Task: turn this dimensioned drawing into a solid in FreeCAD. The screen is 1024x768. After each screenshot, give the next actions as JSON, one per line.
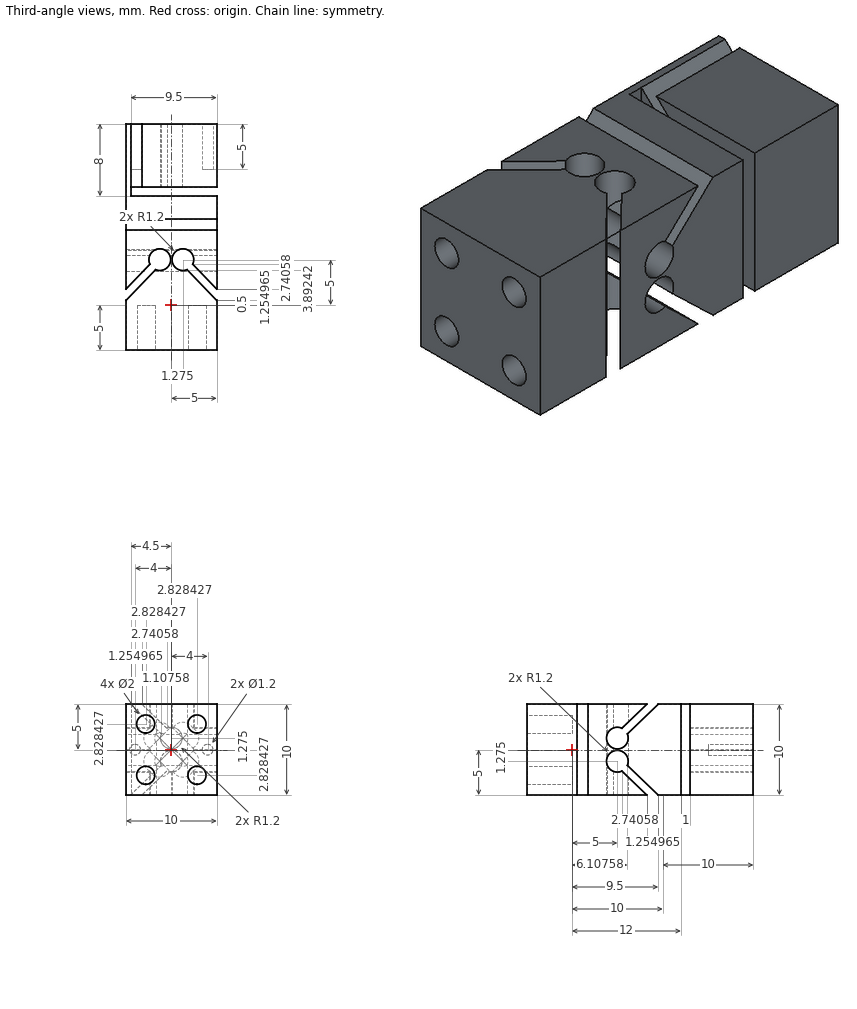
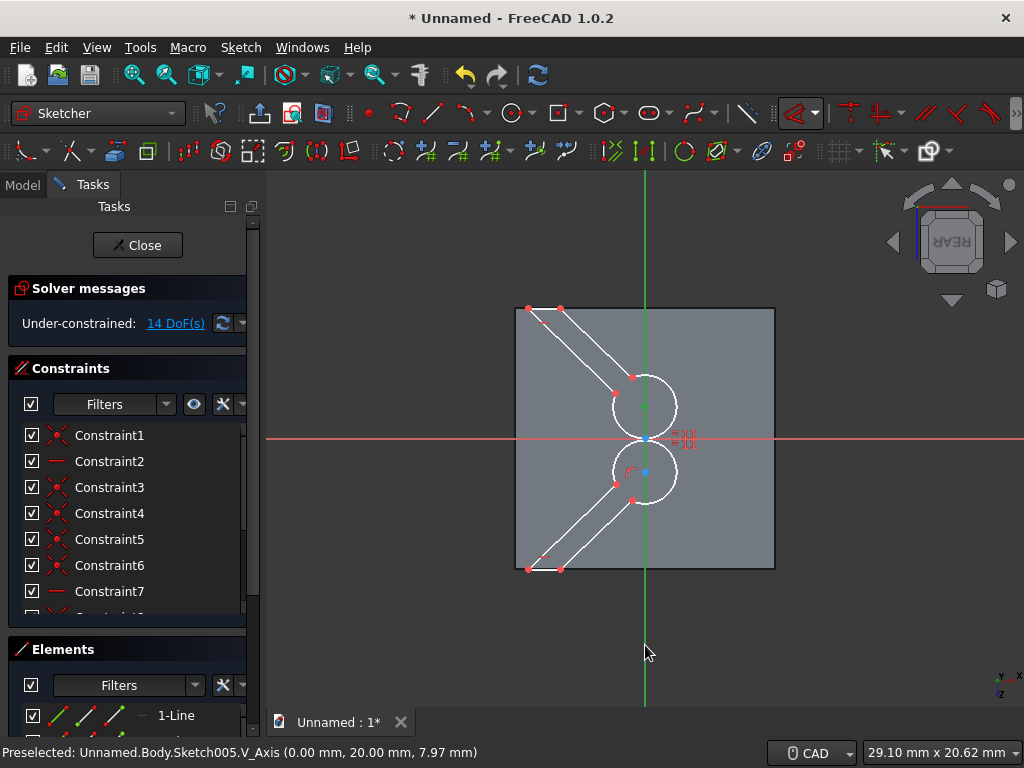
{"action": "left_click", "coordinate": [850, 114]}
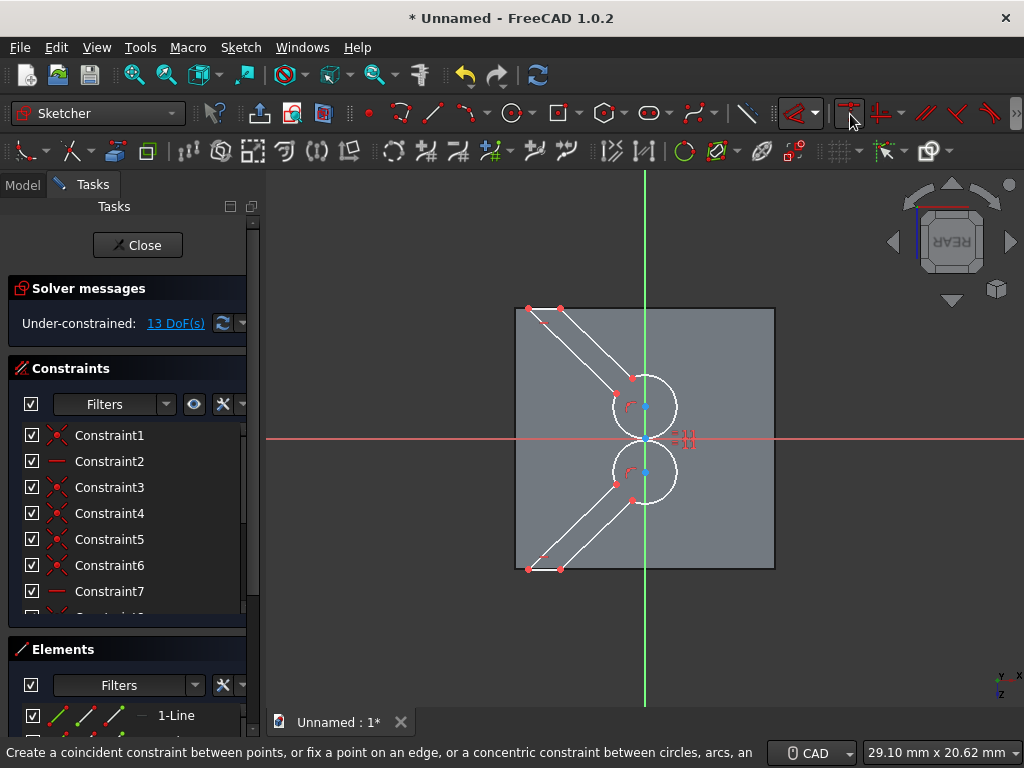
{"action": "left_click", "coordinate": [632, 501]}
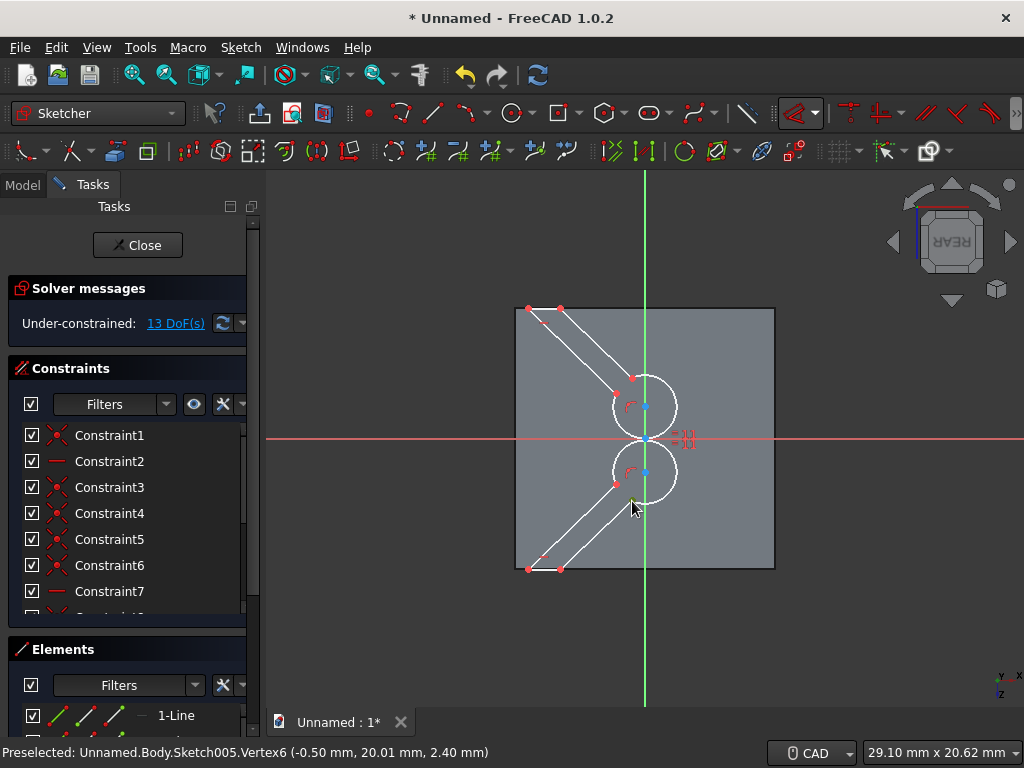
{"action": "left_click", "coordinate": [632, 378]}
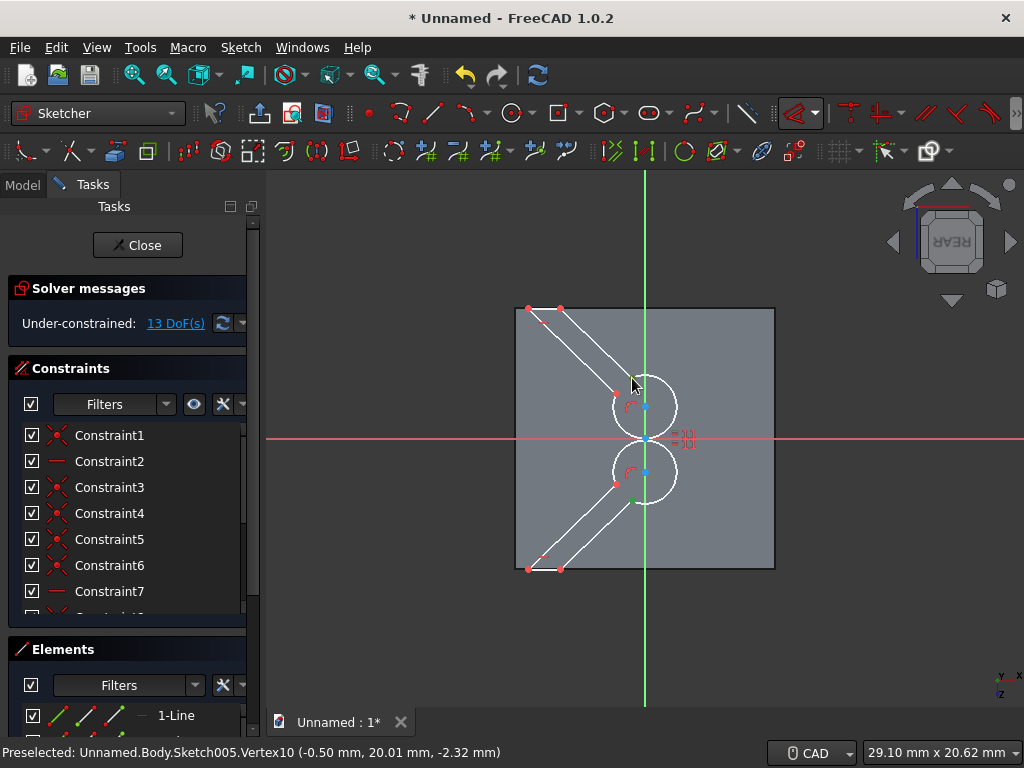
{"action": "left_click", "coordinate": [334, 438]}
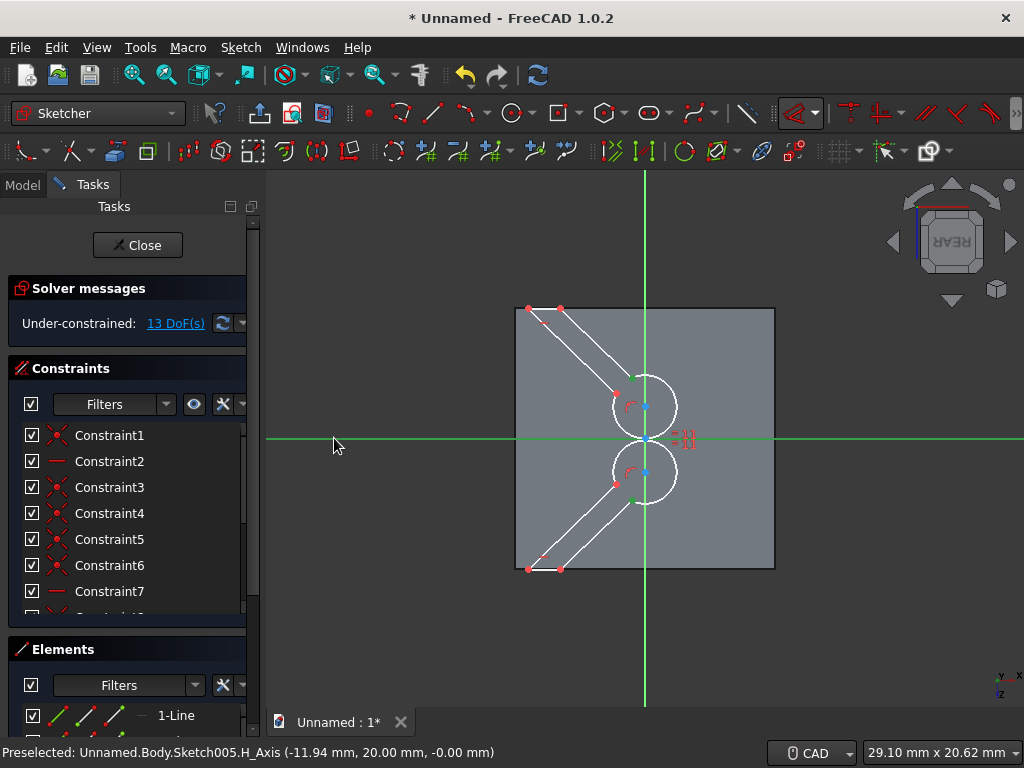
{"action": "key", "text": "s"}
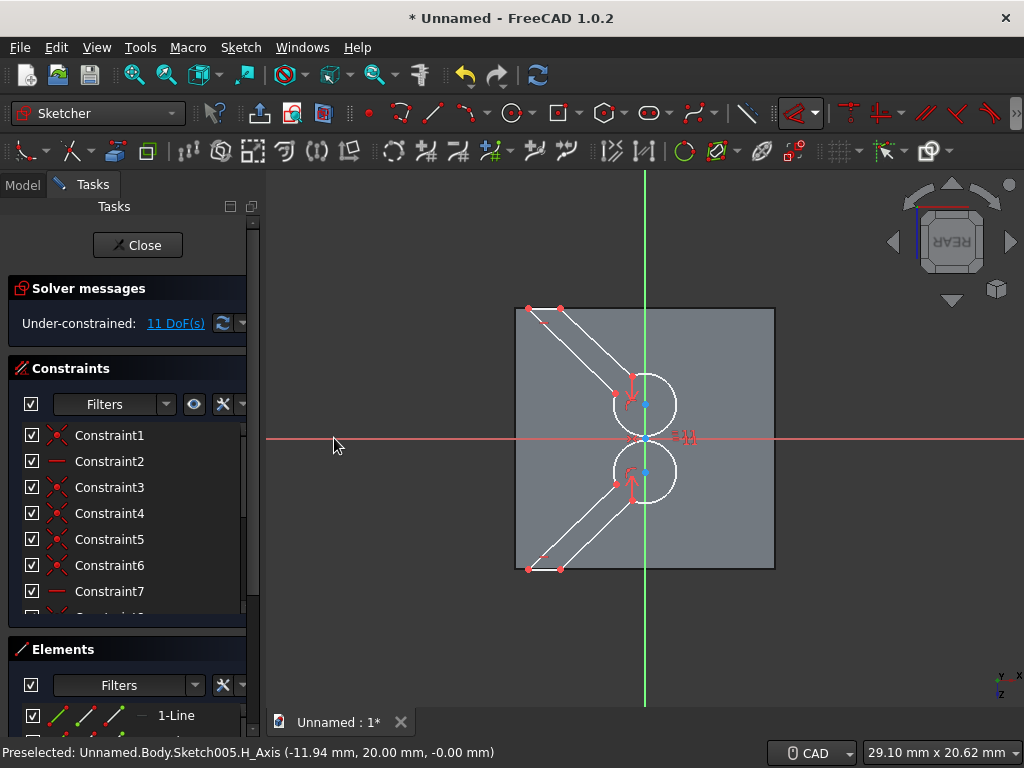
{"action": "left_click", "coordinate": [560, 570]}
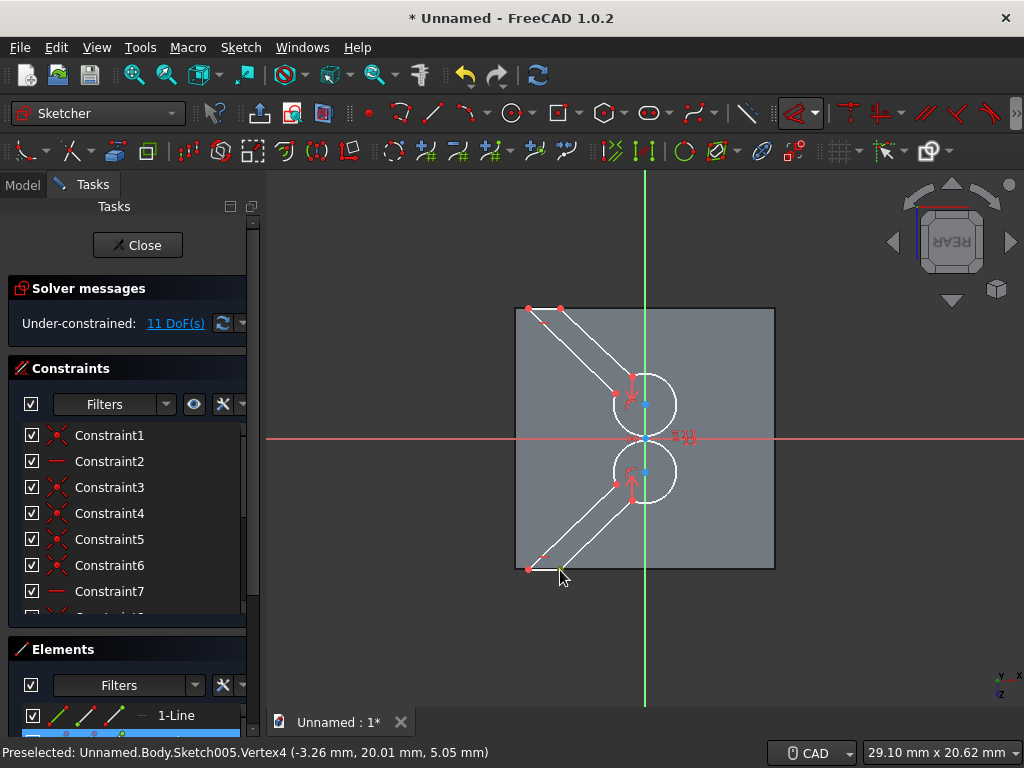
{"action": "left_click", "coordinate": [560, 309]}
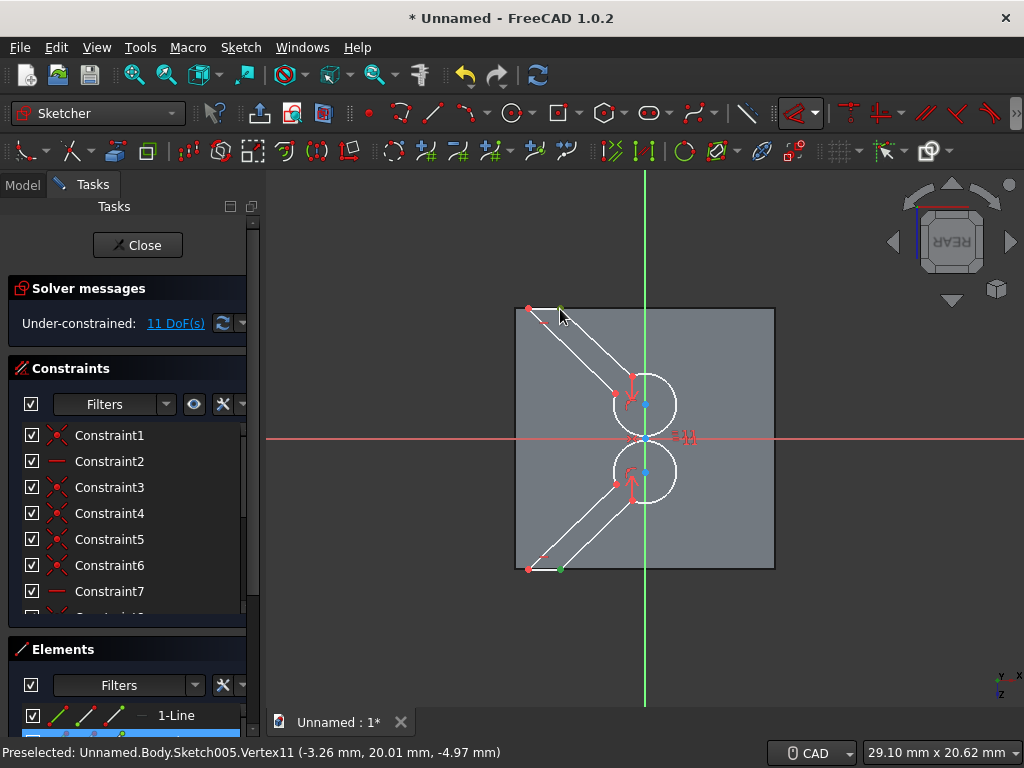
{"action": "left_click", "coordinate": [334, 438]}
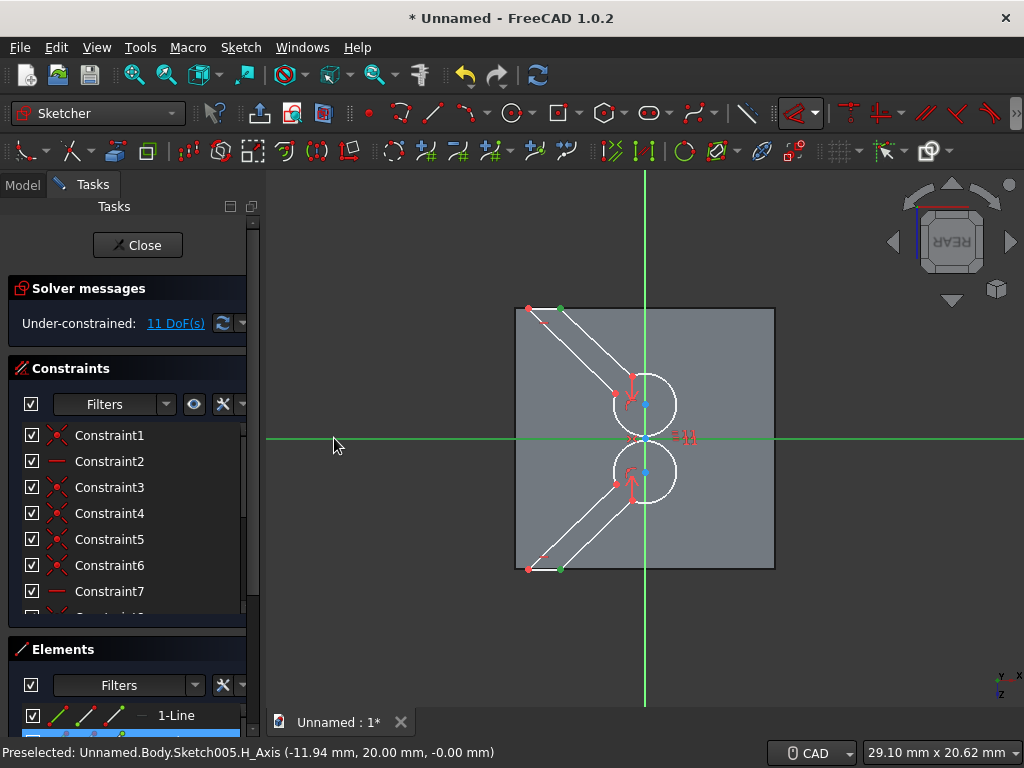
{"action": "key", "text": "s"}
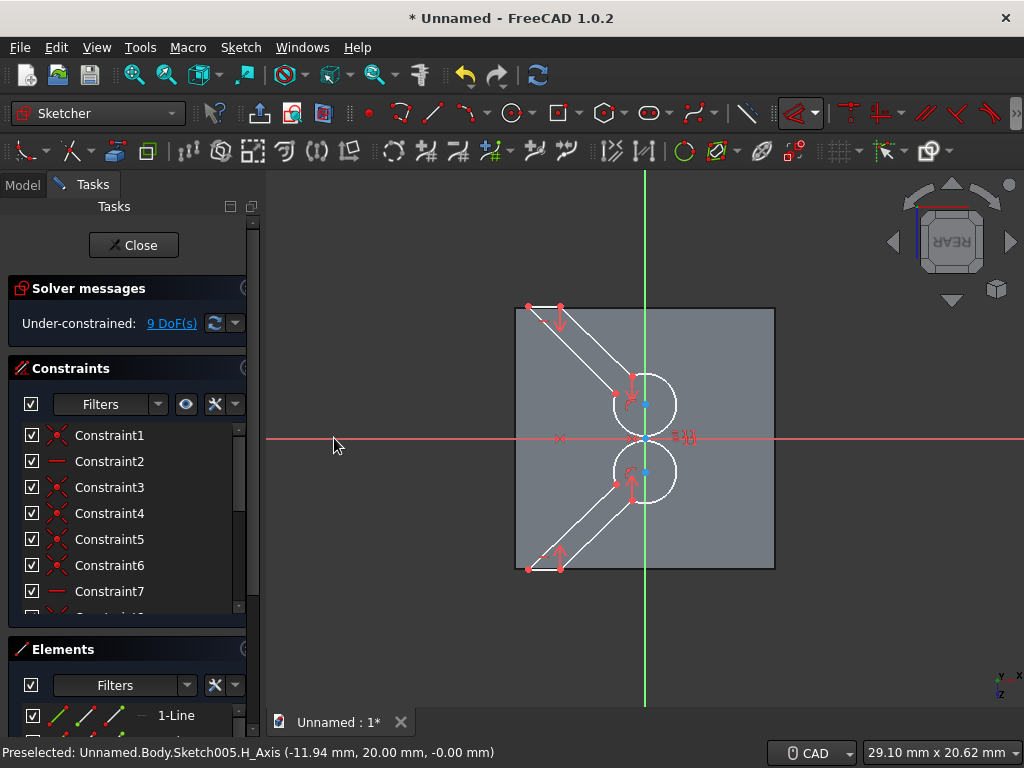
{"action": "scroll", "coordinate": [675, 482], "scroll_direction": "up", "scroll_amount": 2}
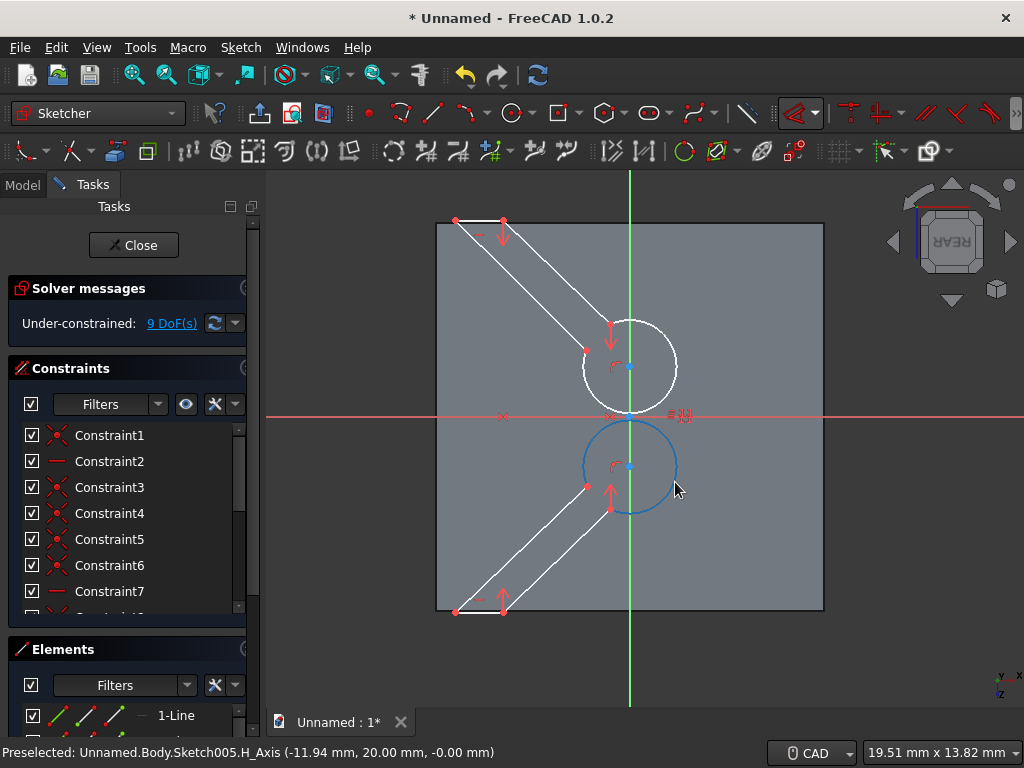
{"action": "left_click", "coordinate": [674, 482]}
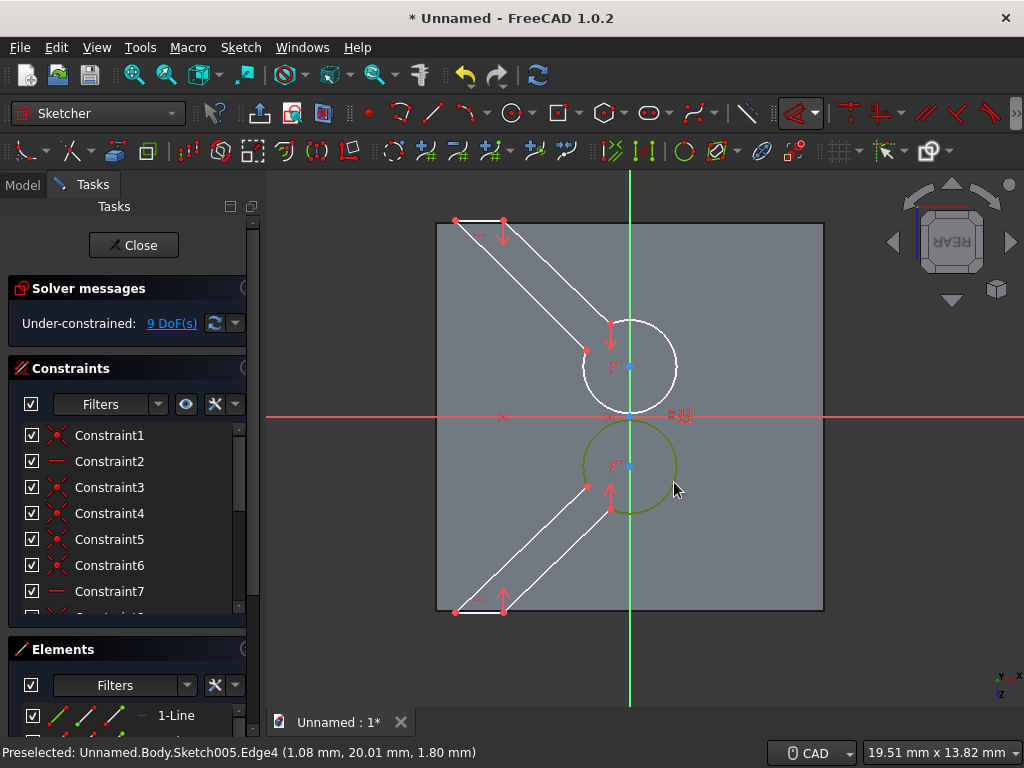
{"action": "left_click", "coordinate": [818, 114]}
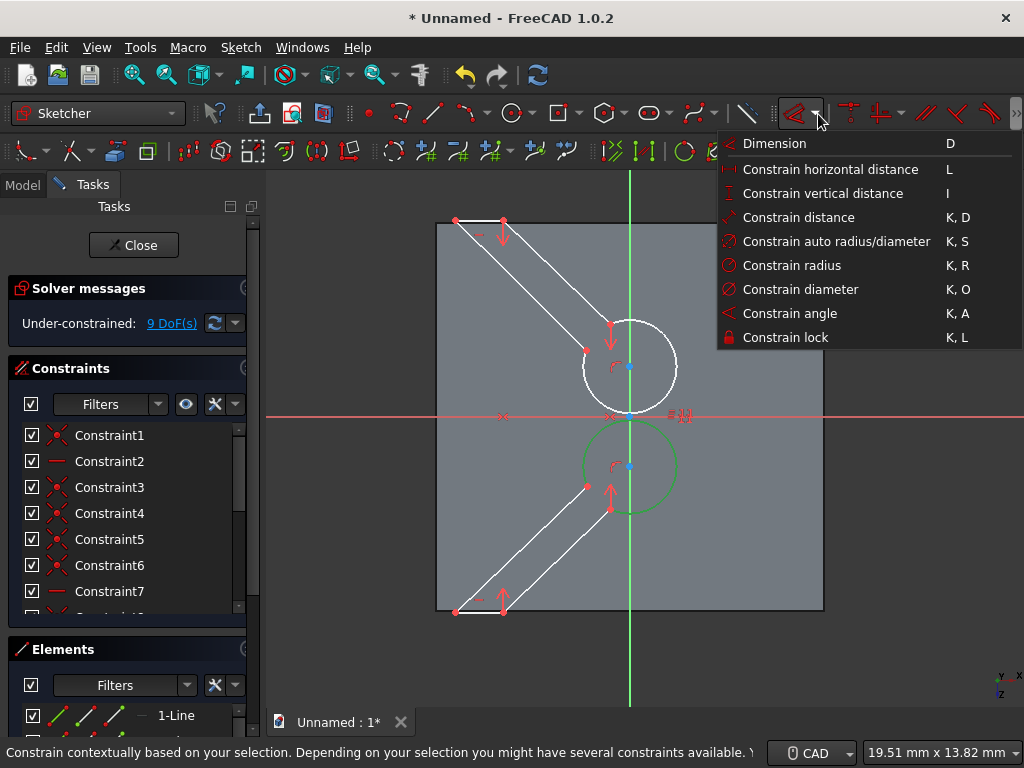
{"action": "left_click", "coordinate": [870, 265]}